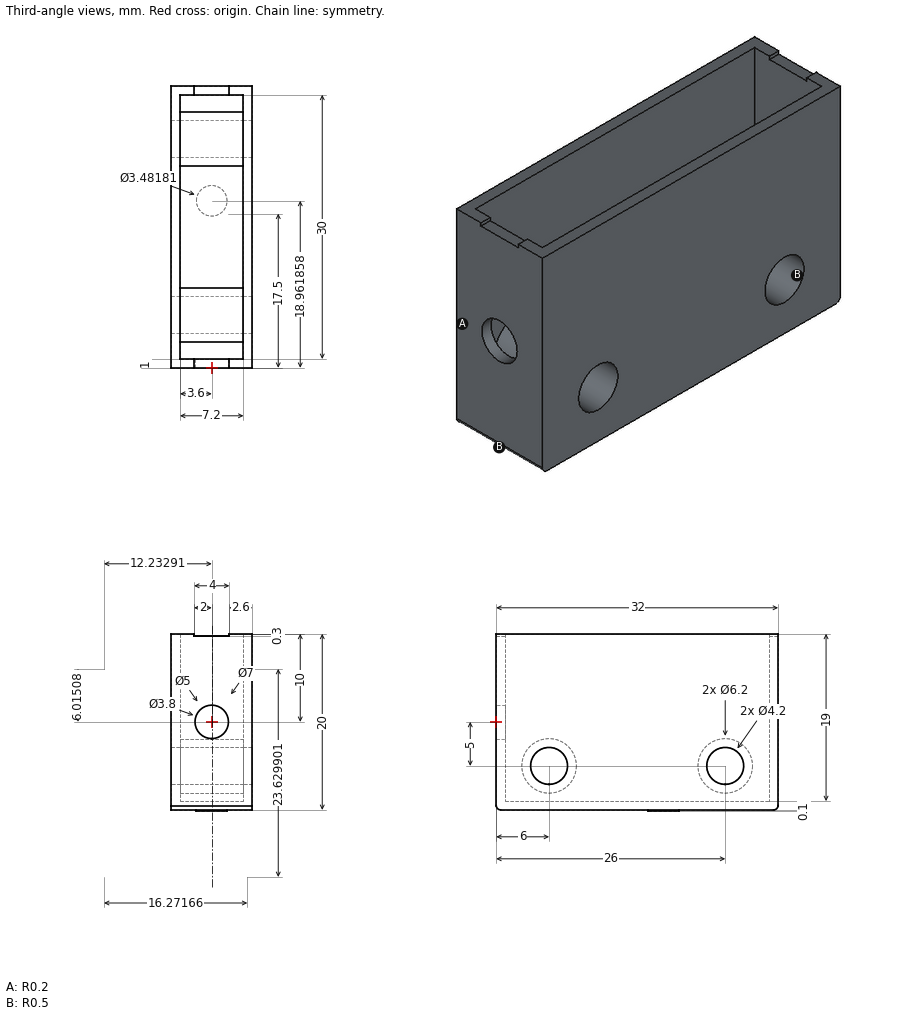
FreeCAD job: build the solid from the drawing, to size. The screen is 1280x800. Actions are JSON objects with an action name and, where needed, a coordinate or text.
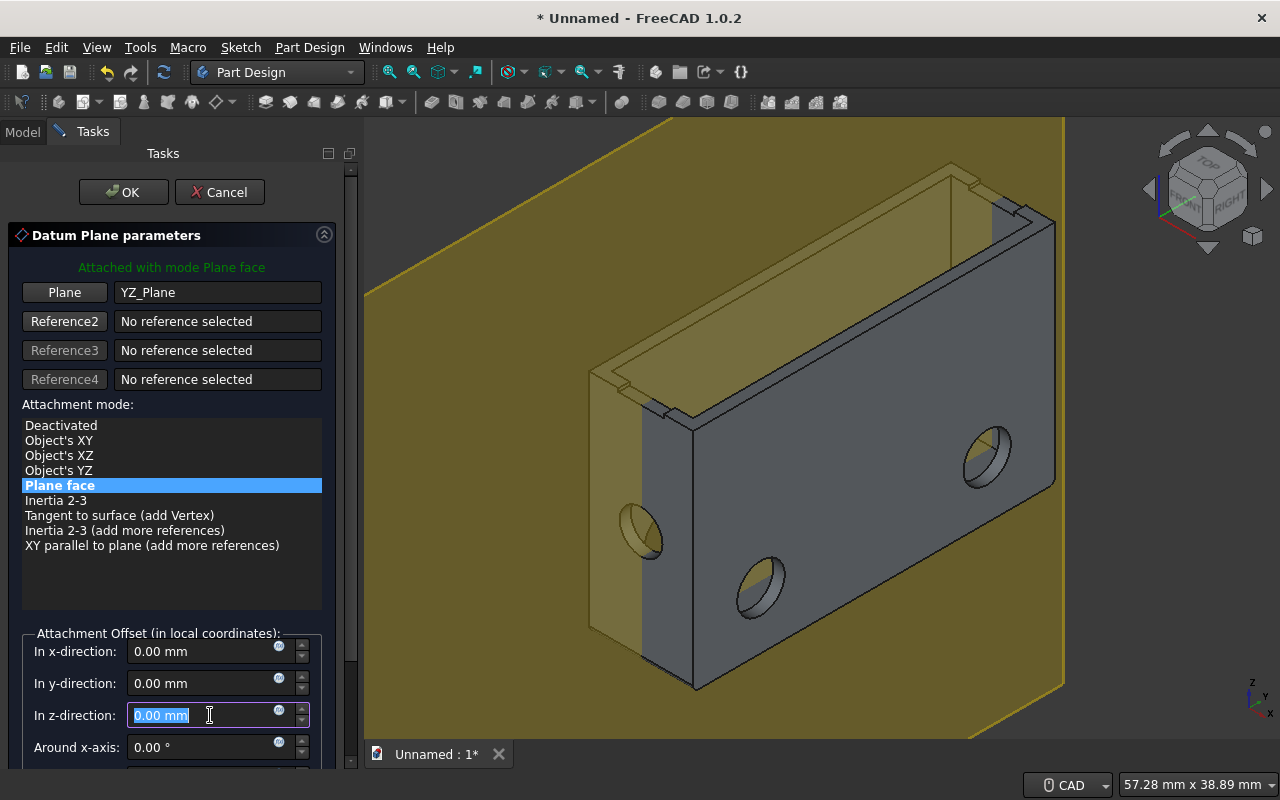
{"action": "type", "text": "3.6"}
{"action": "key", "text": "Tab"}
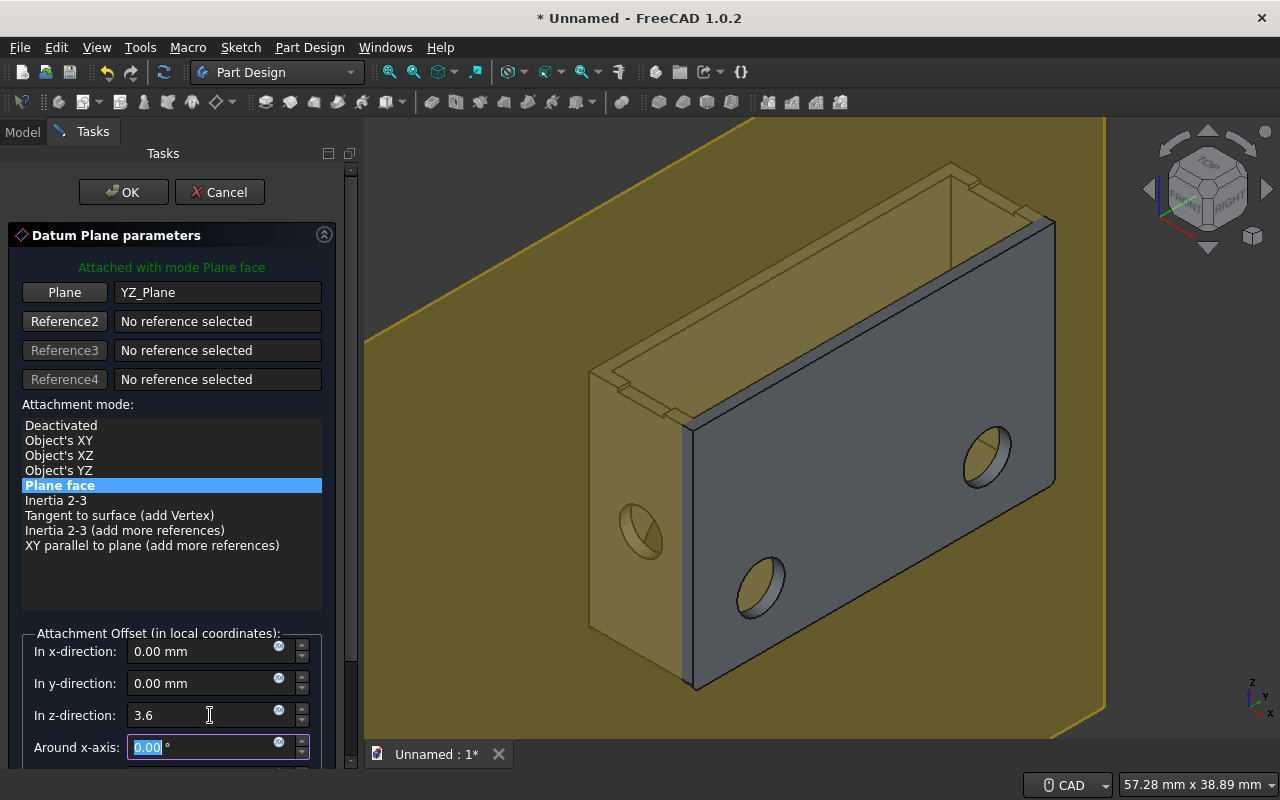
{"action": "left_click", "coordinate": [124, 192]}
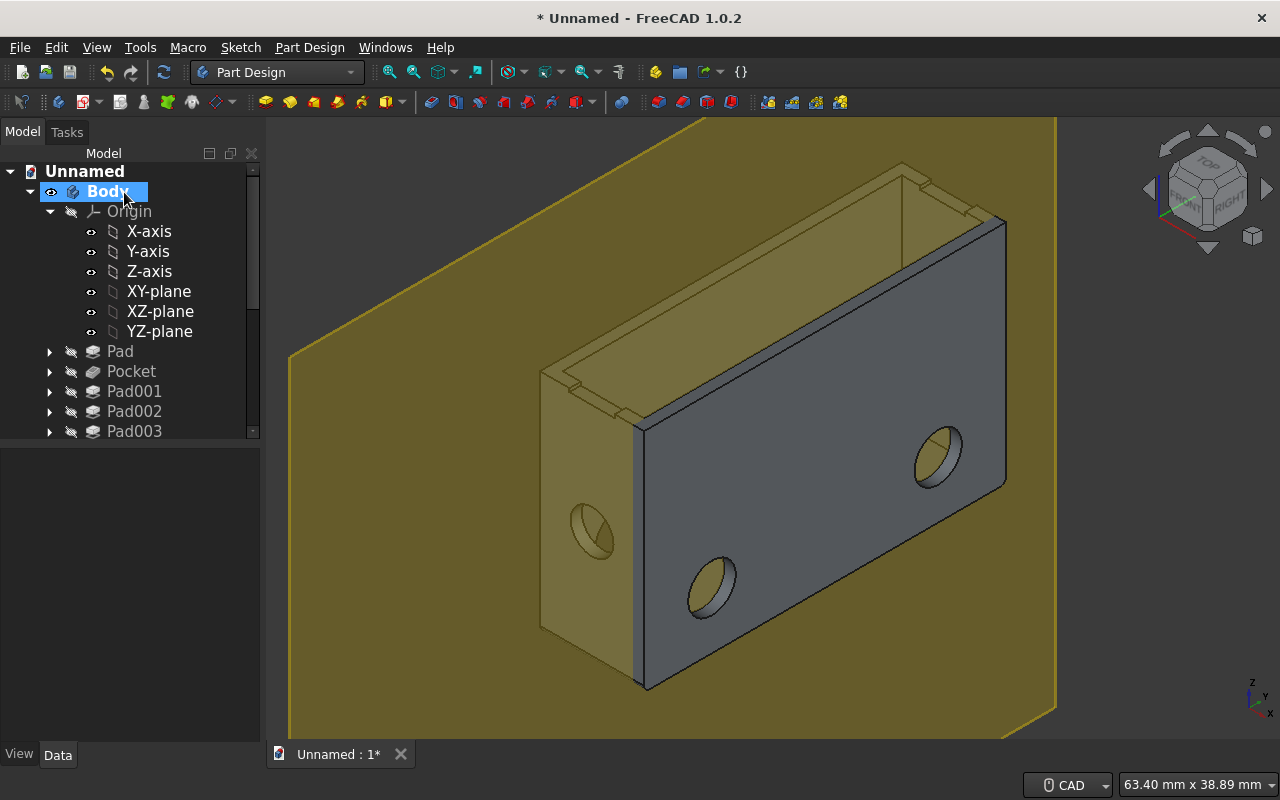
{"action": "scroll", "coordinate": [100, 307], "scroll_direction": "down", "scroll_amount": 3}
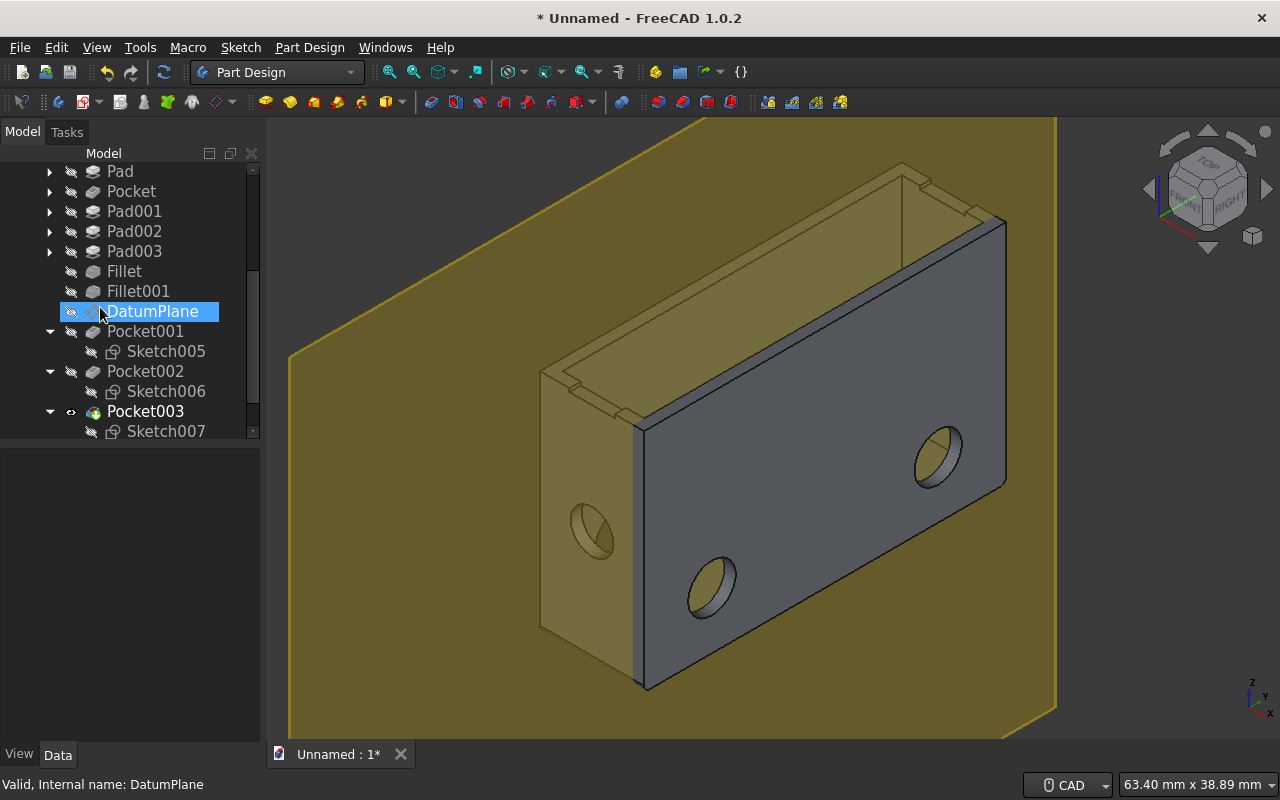
{"action": "scroll", "coordinate": [140, 307], "scroll_direction": "up", "scroll_amount": 15}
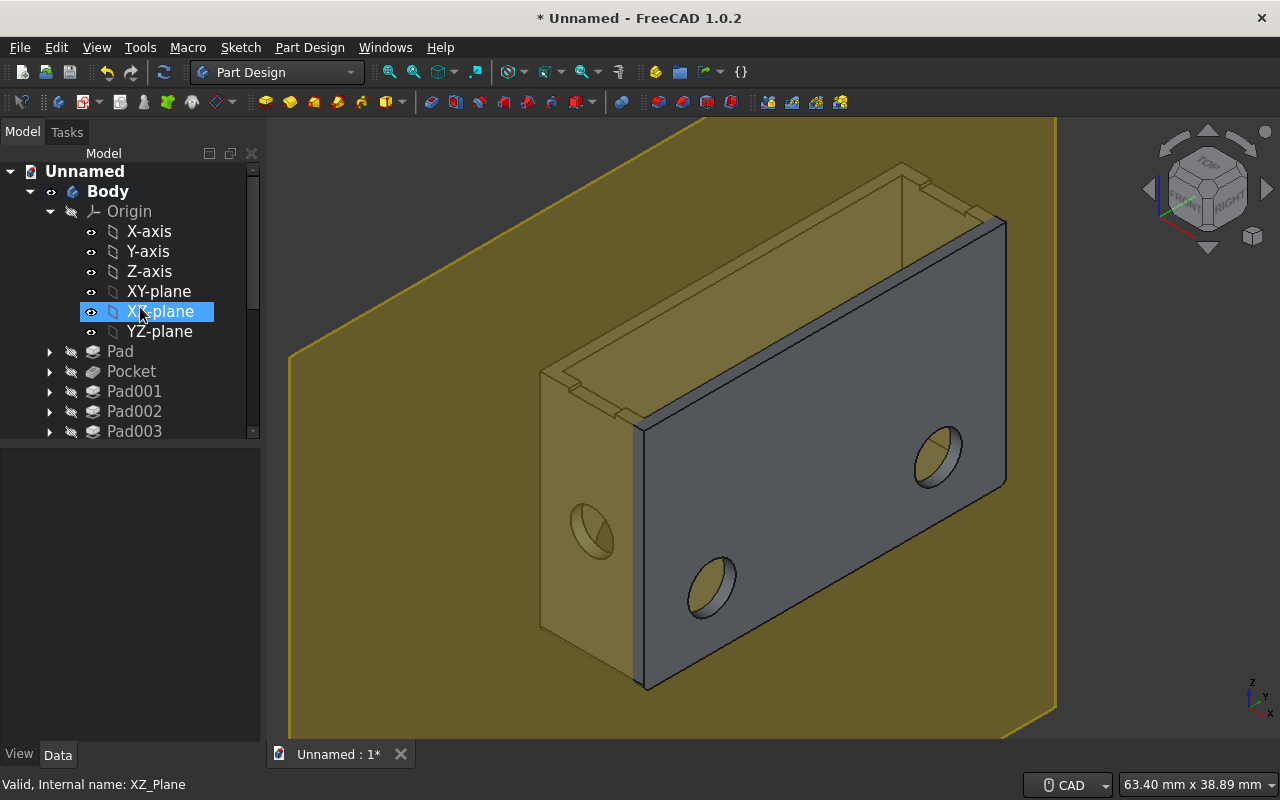
{"action": "scroll", "coordinate": [100, 307], "scroll_direction": "down", "scroll_amount": 6}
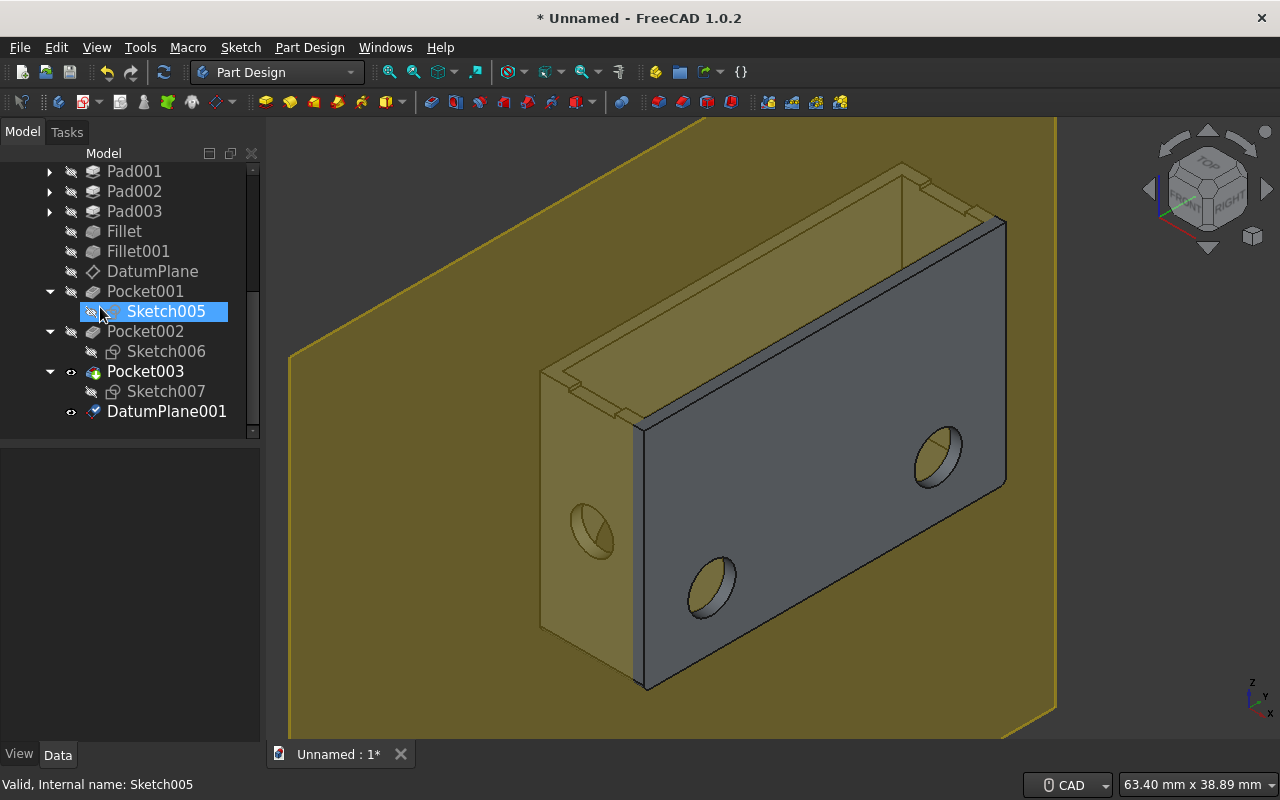
{"action": "left_click", "coordinate": [116, 412]}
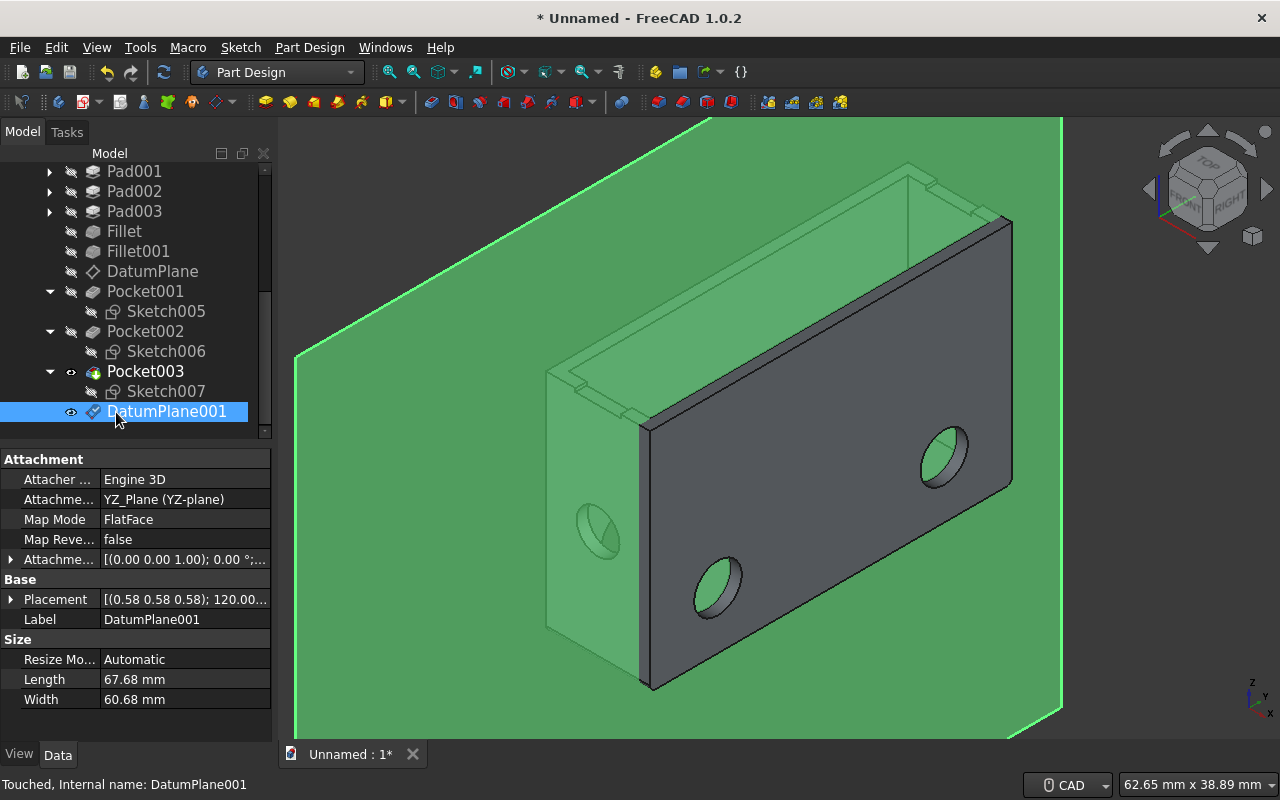
{"action": "left_click", "coordinate": [84, 102]}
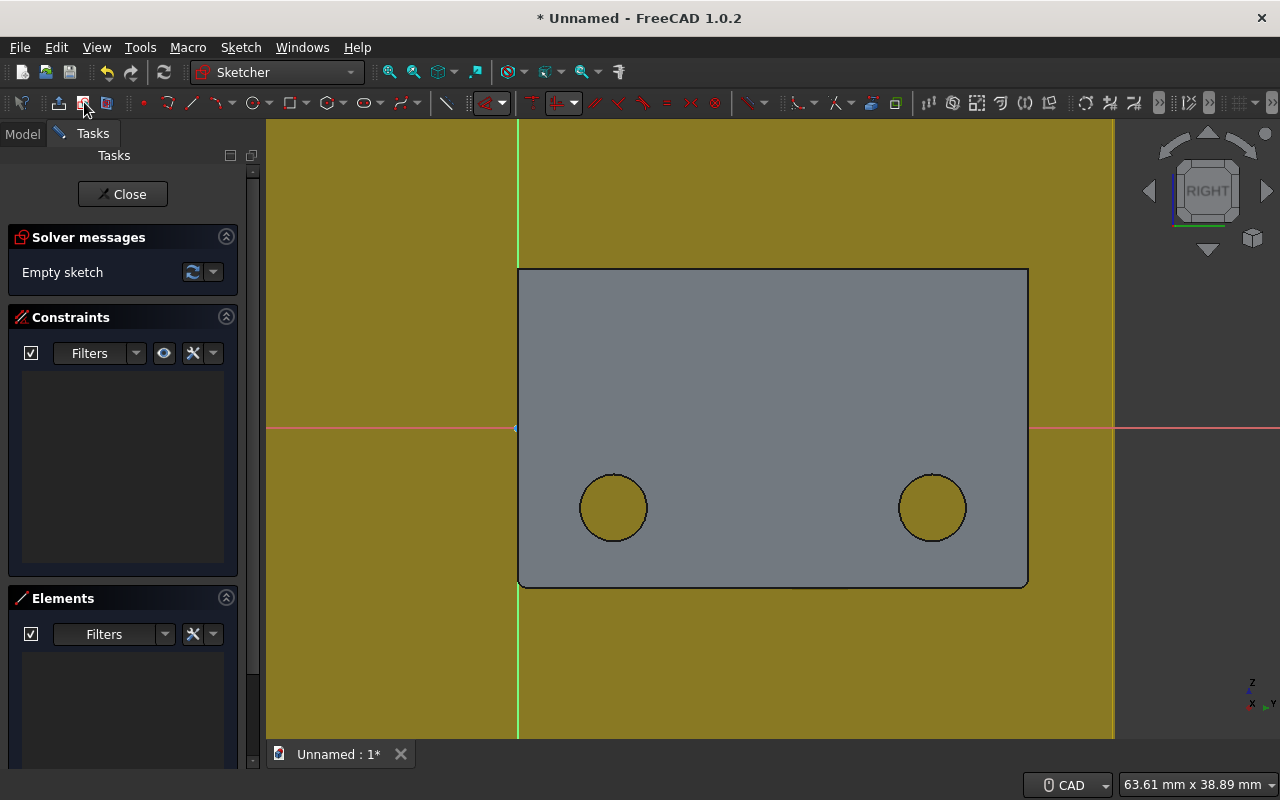
{"action": "left_click", "coordinate": [108, 104]}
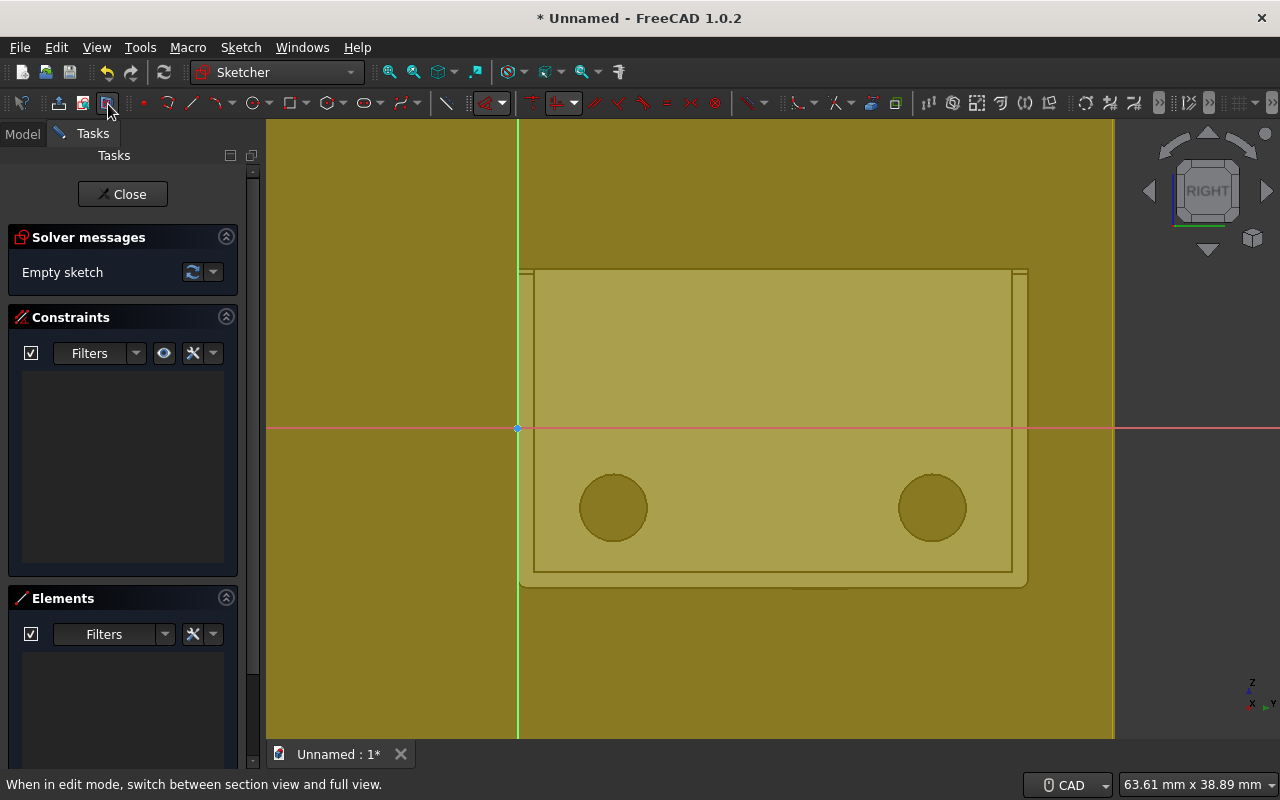
{"action": "left_click", "coordinate": [254, 104]}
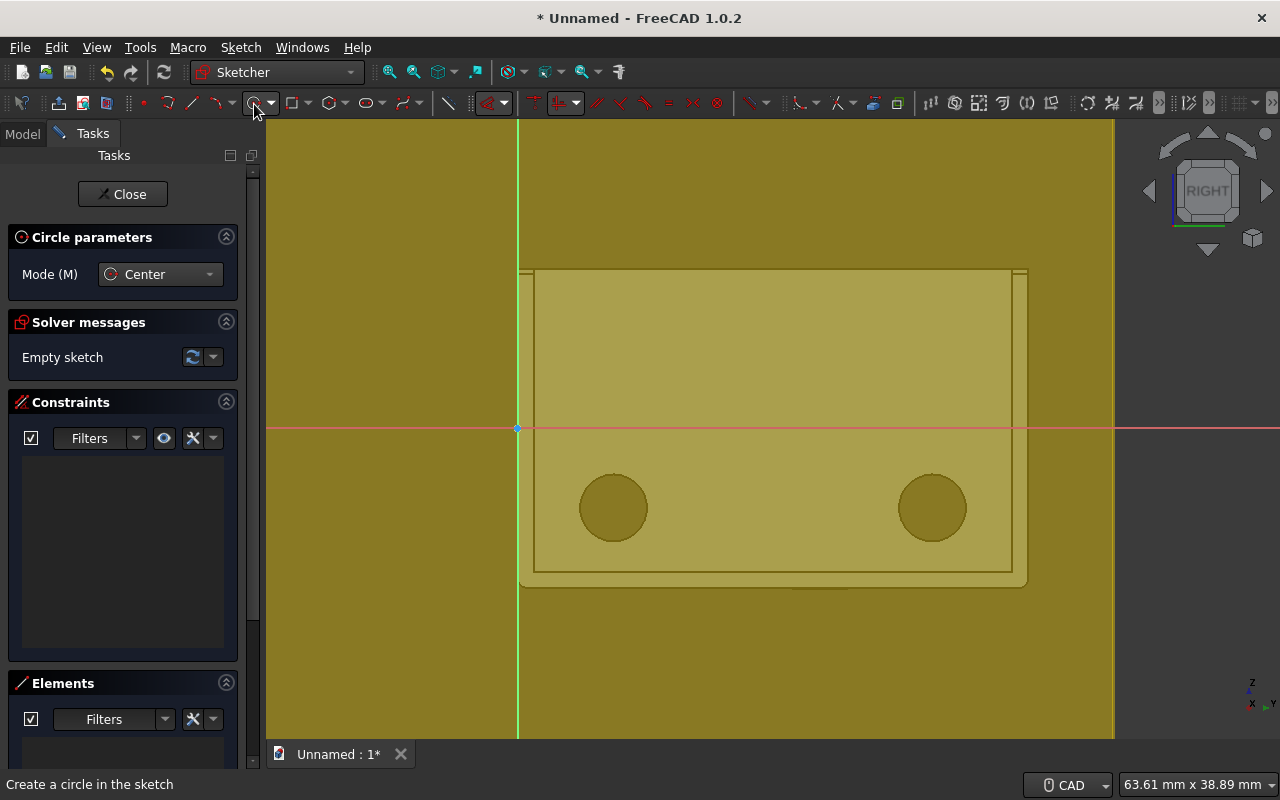
{"action": "left_click", "coordinate": [932, 508]}
{"action": "mouse_move", "coordinate": [967, 473]}